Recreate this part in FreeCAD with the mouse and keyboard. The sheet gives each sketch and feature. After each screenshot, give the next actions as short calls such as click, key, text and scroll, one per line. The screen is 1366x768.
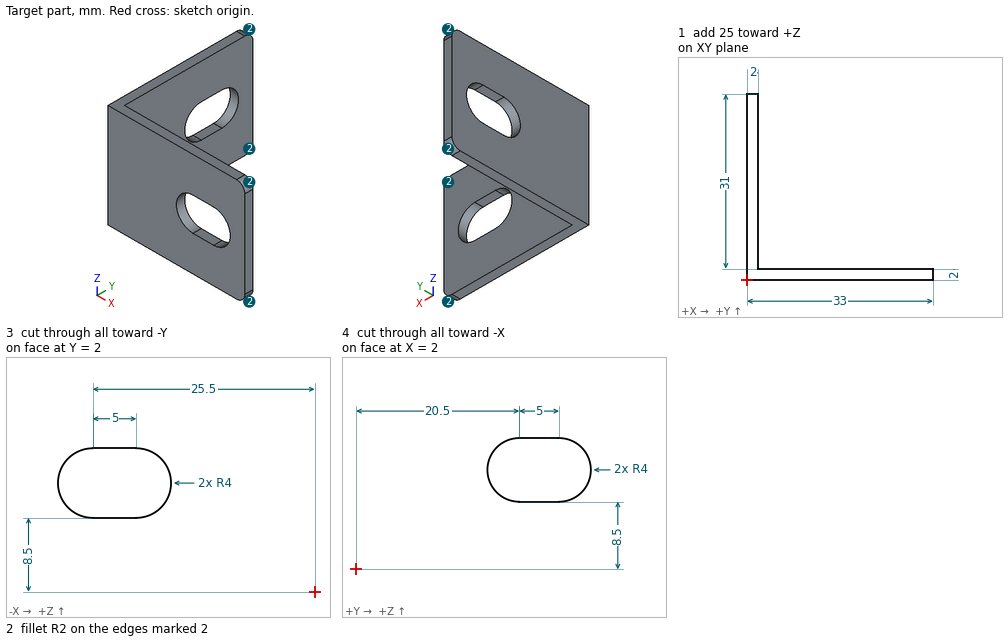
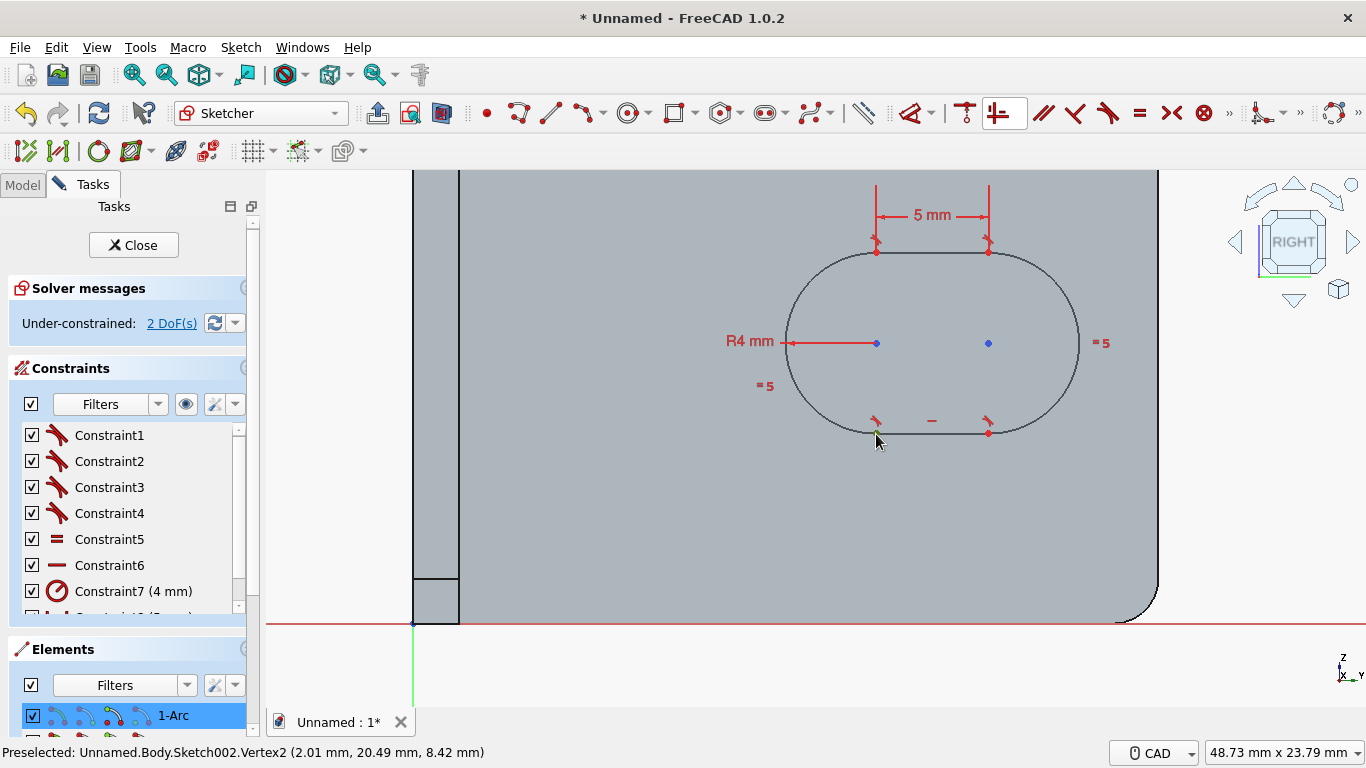
key(i)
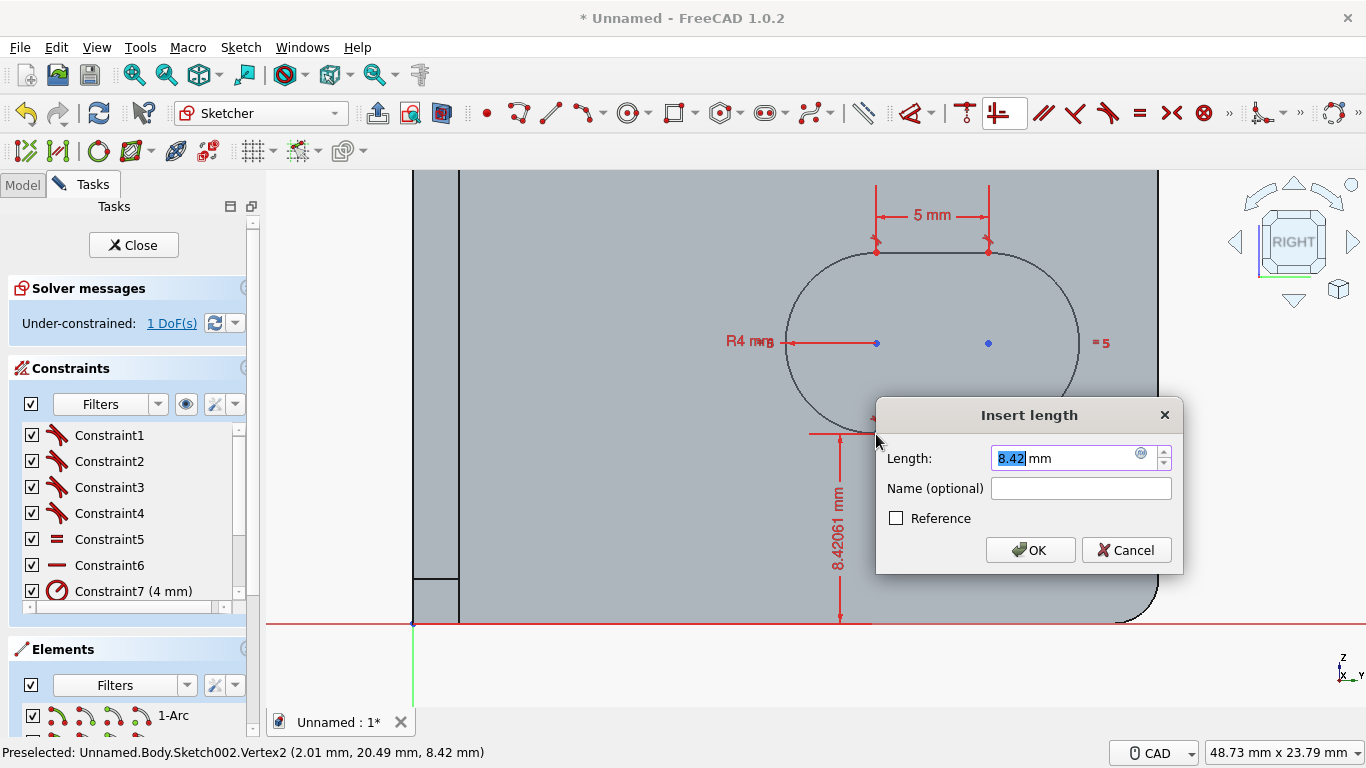
text(8.5)
key(Return)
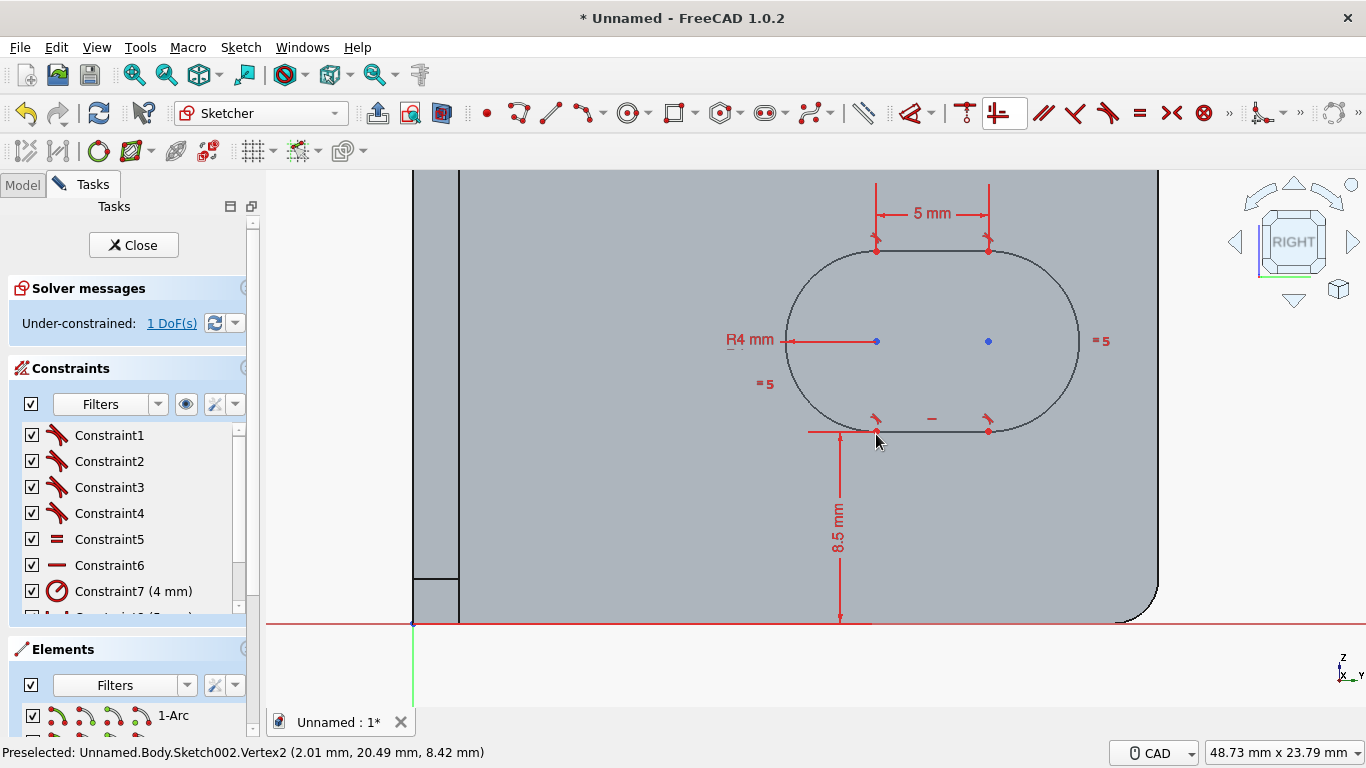
click(876, 251)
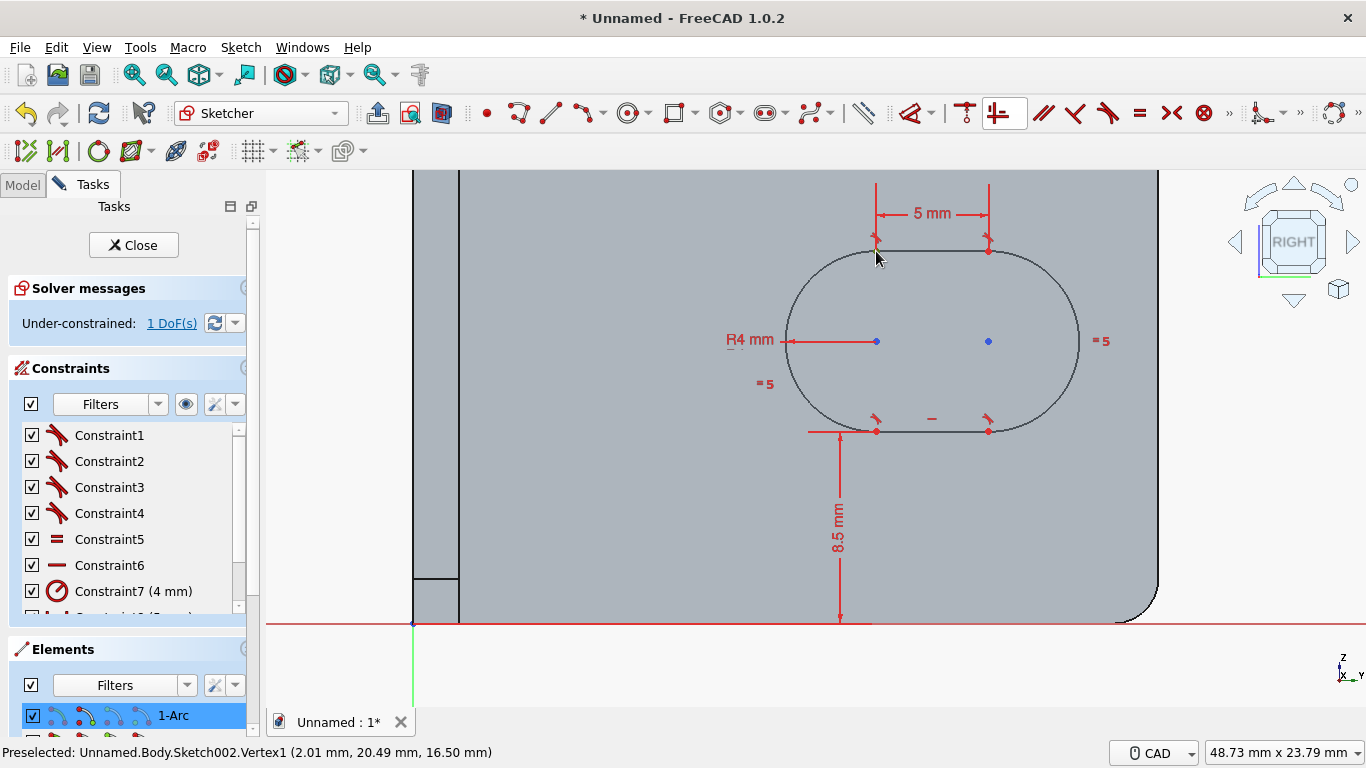
key(l)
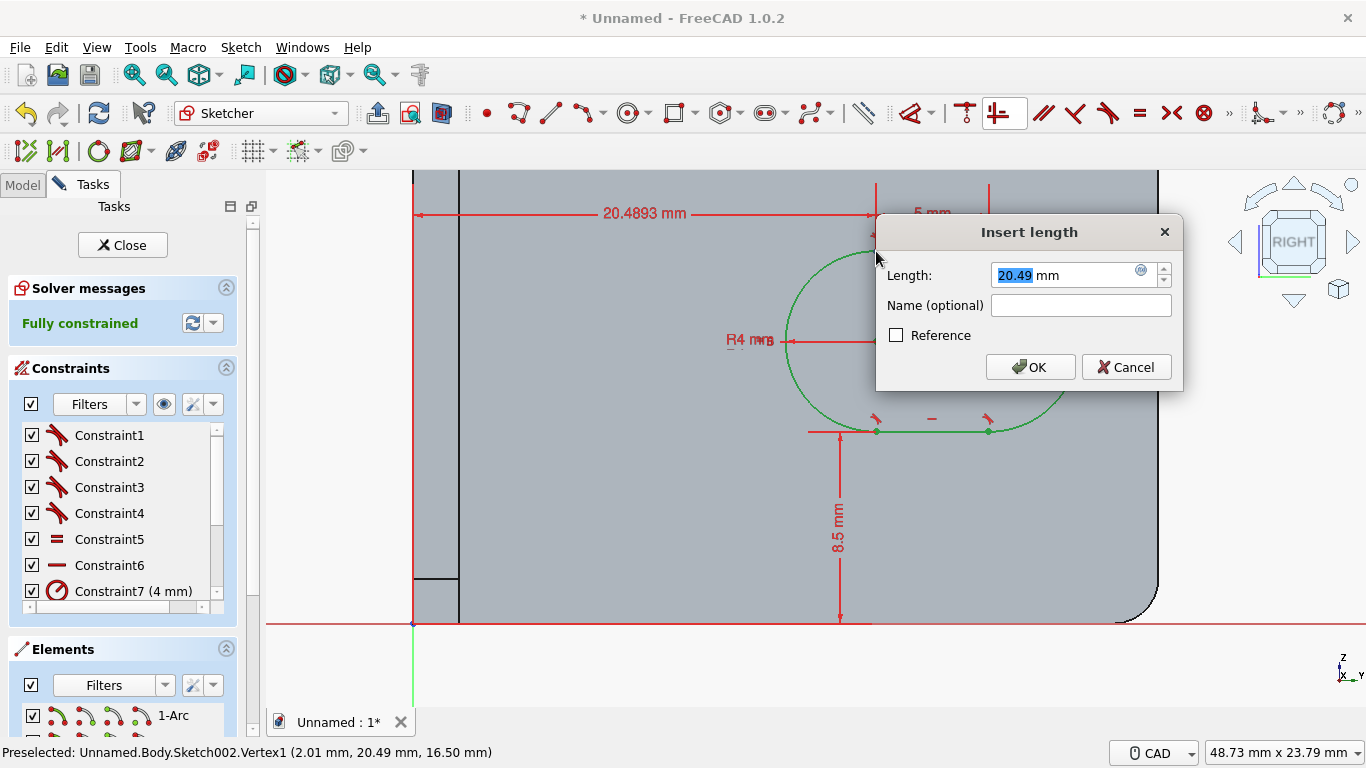
text(20.5)
key(Return)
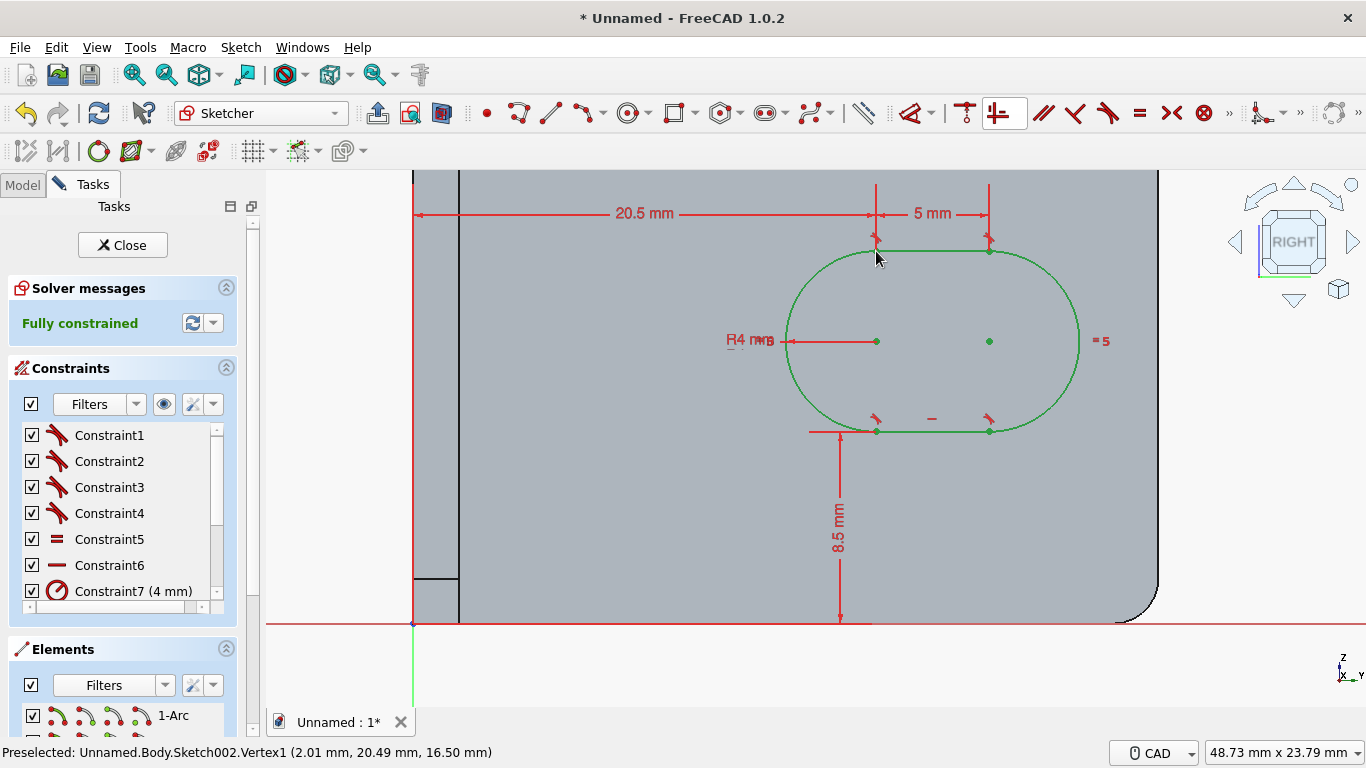
click(123, 245)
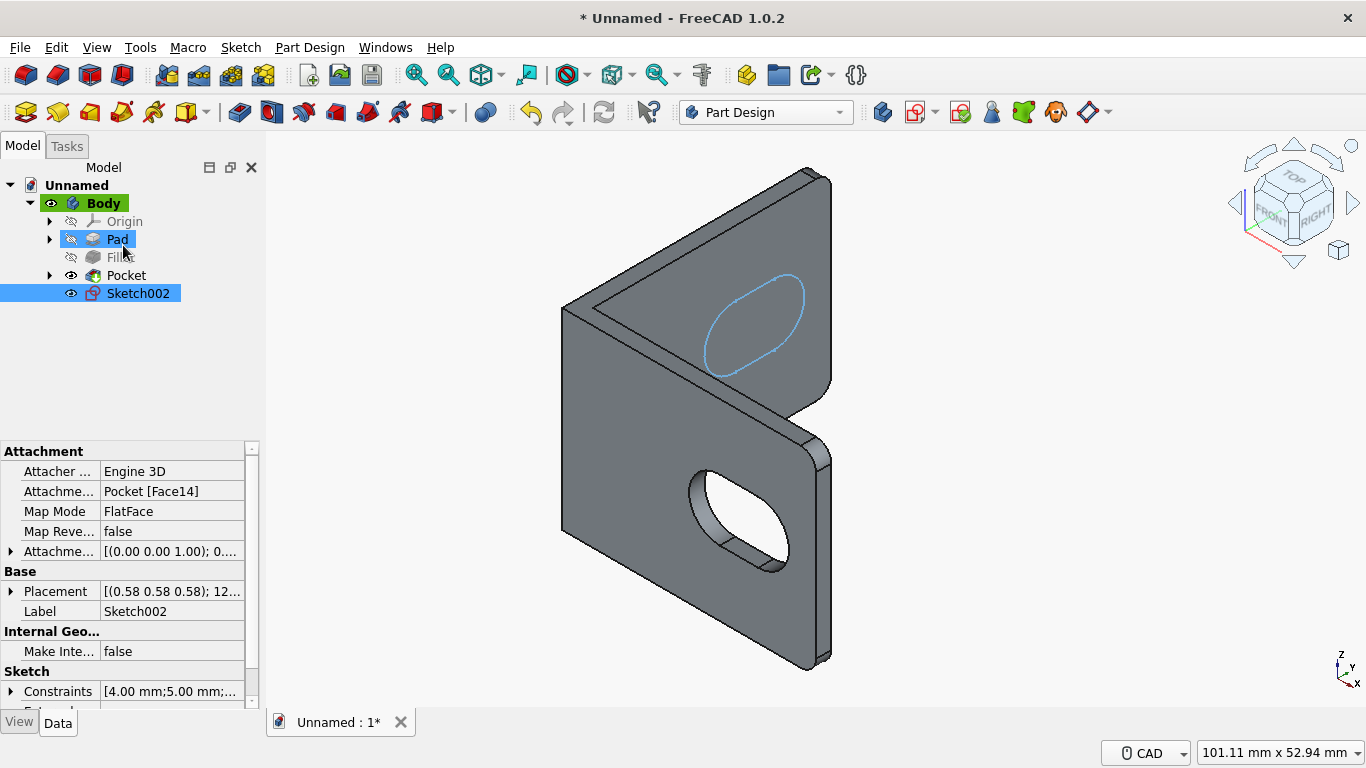
click(240, 112)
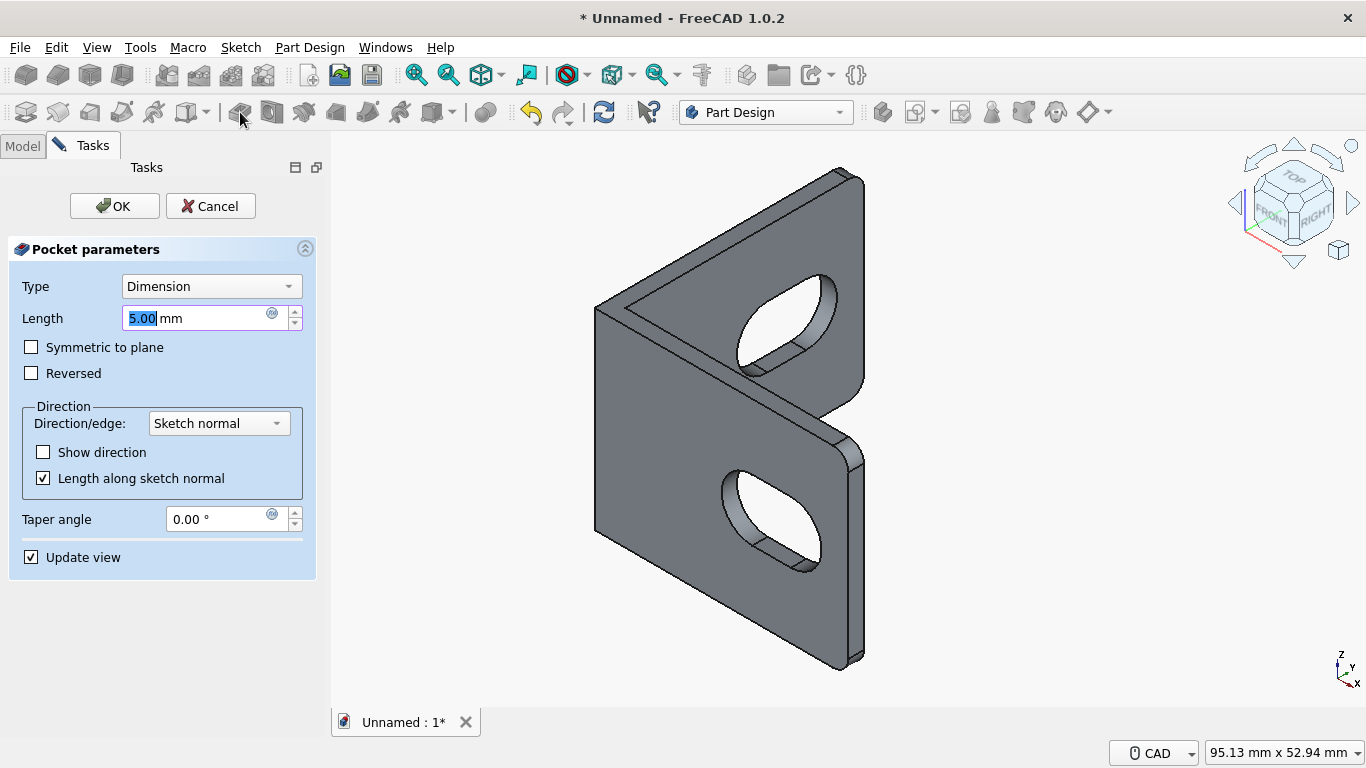
click(212, 286)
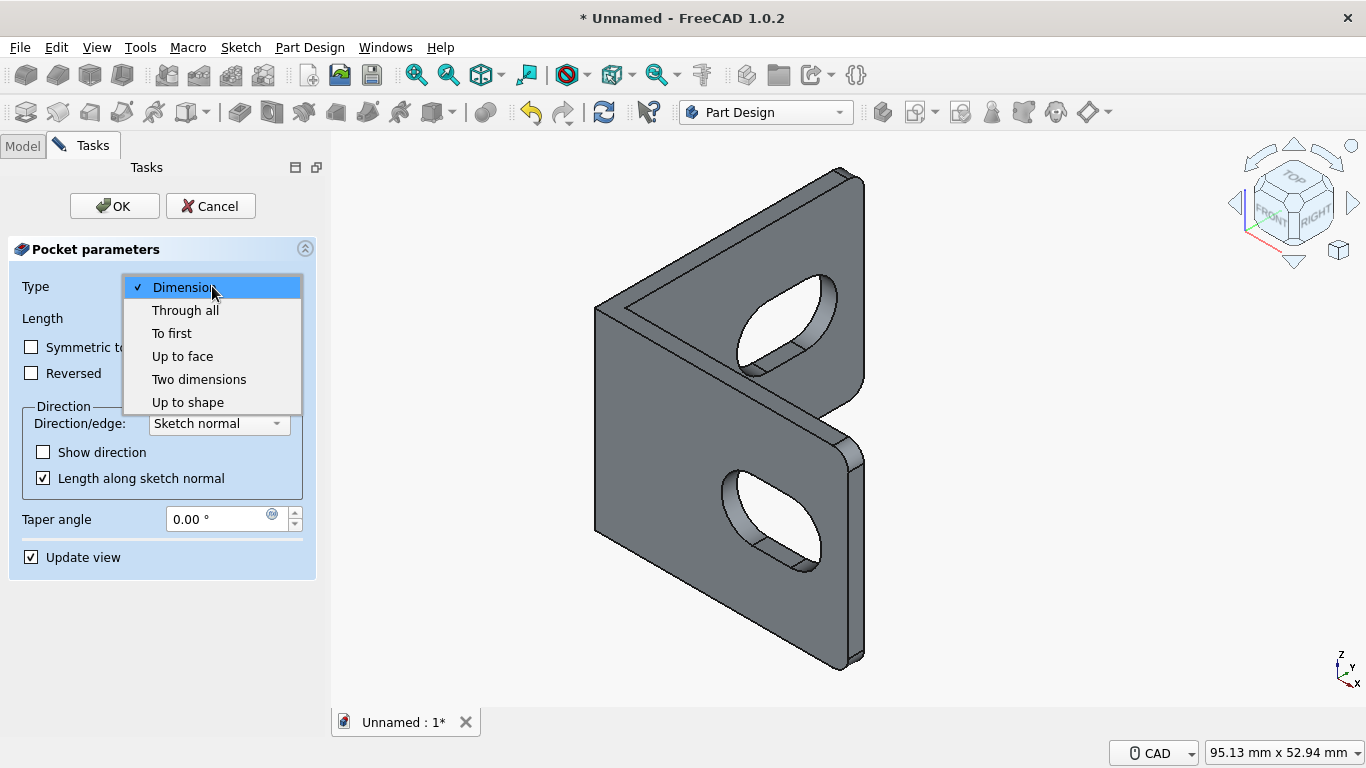
click(212, 310)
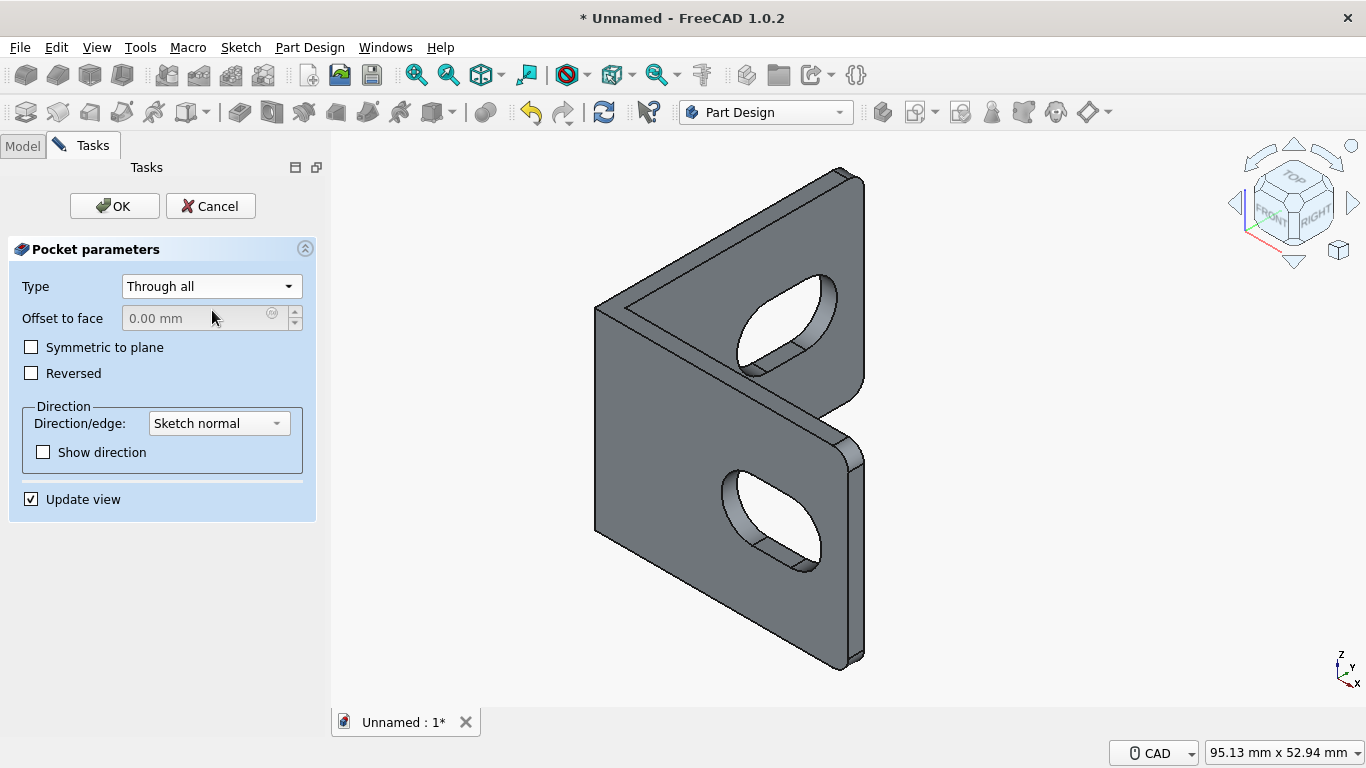
click(115, 206)